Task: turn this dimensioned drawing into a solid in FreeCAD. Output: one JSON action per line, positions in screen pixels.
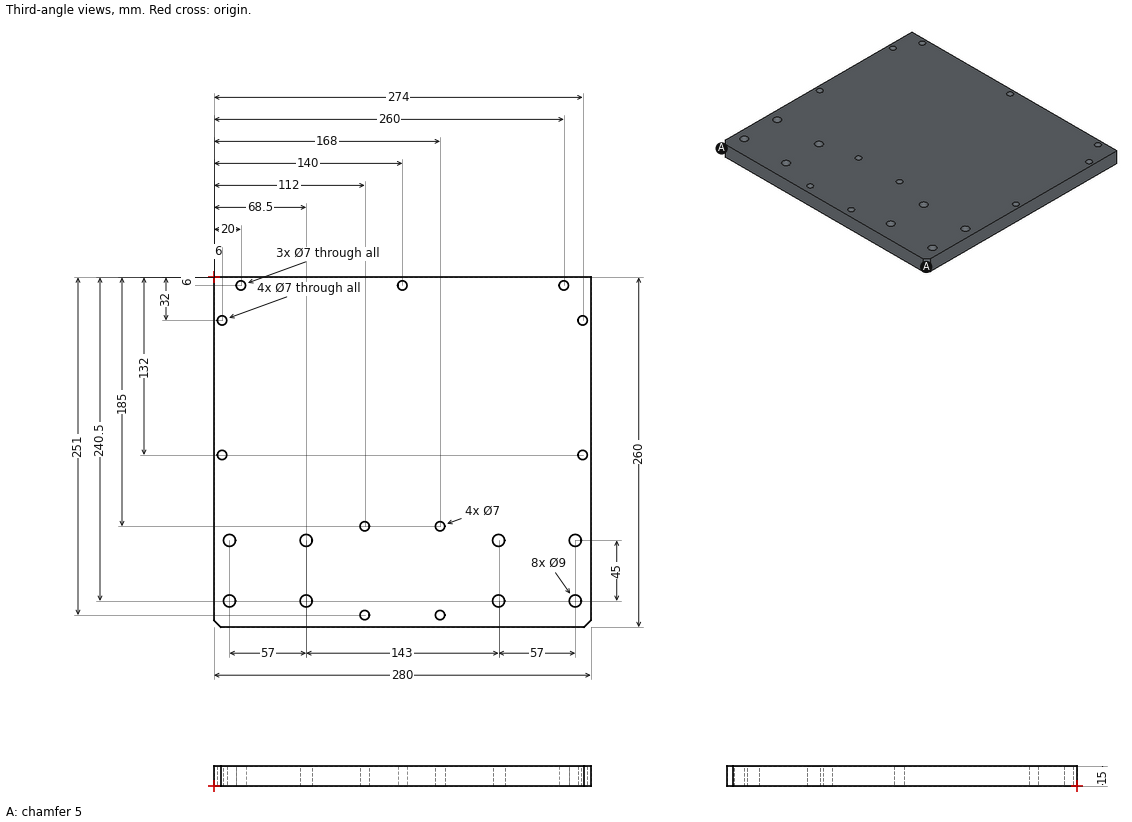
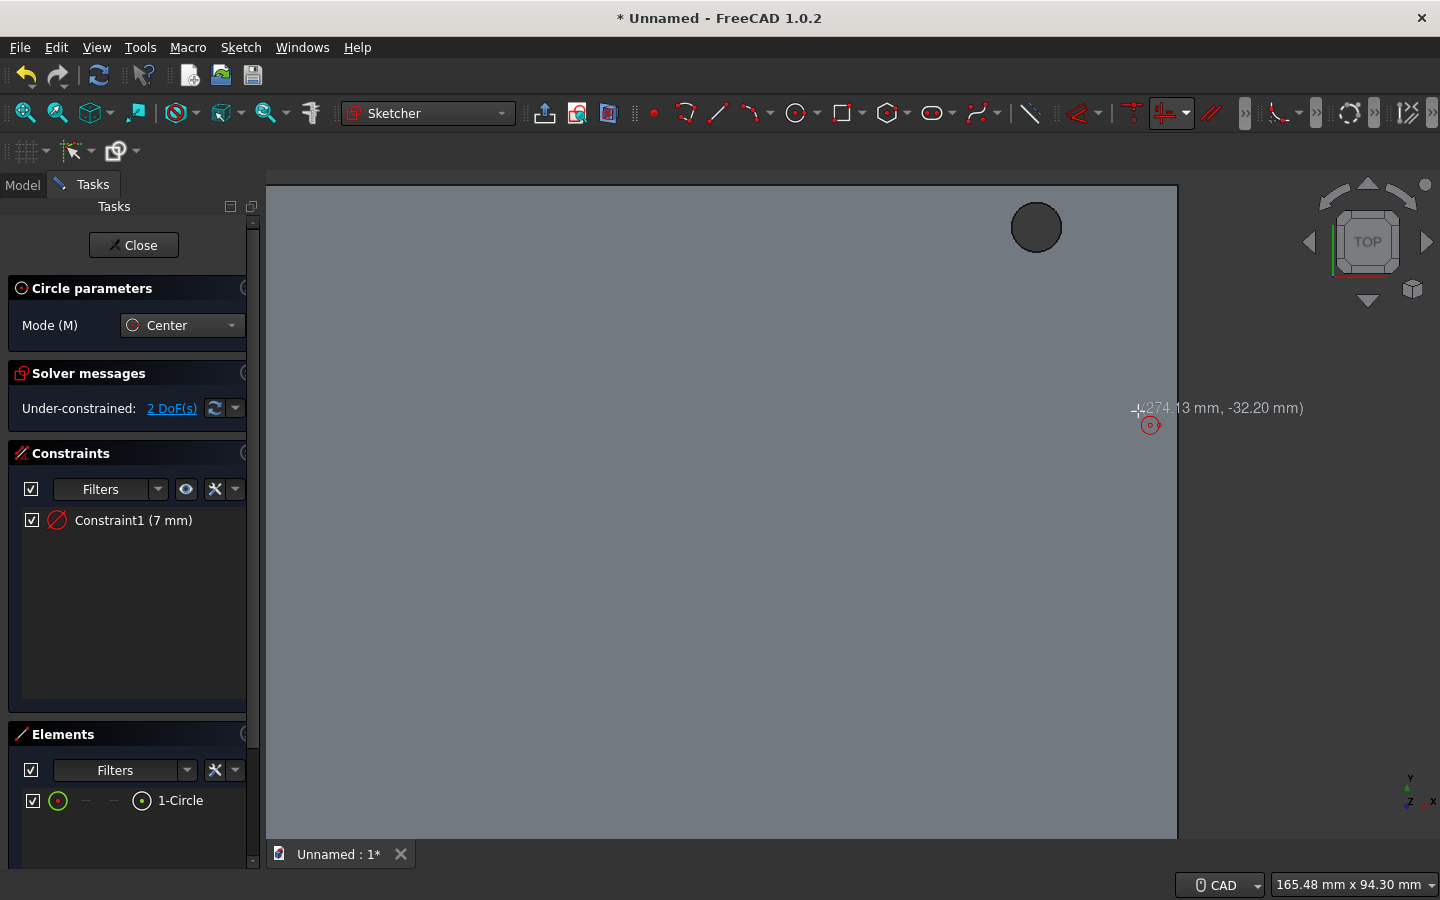
{"action": "left_click", "coordinate": [1136, 412]}
{"action": "mouse_move", "coordinate": [1153, 394]}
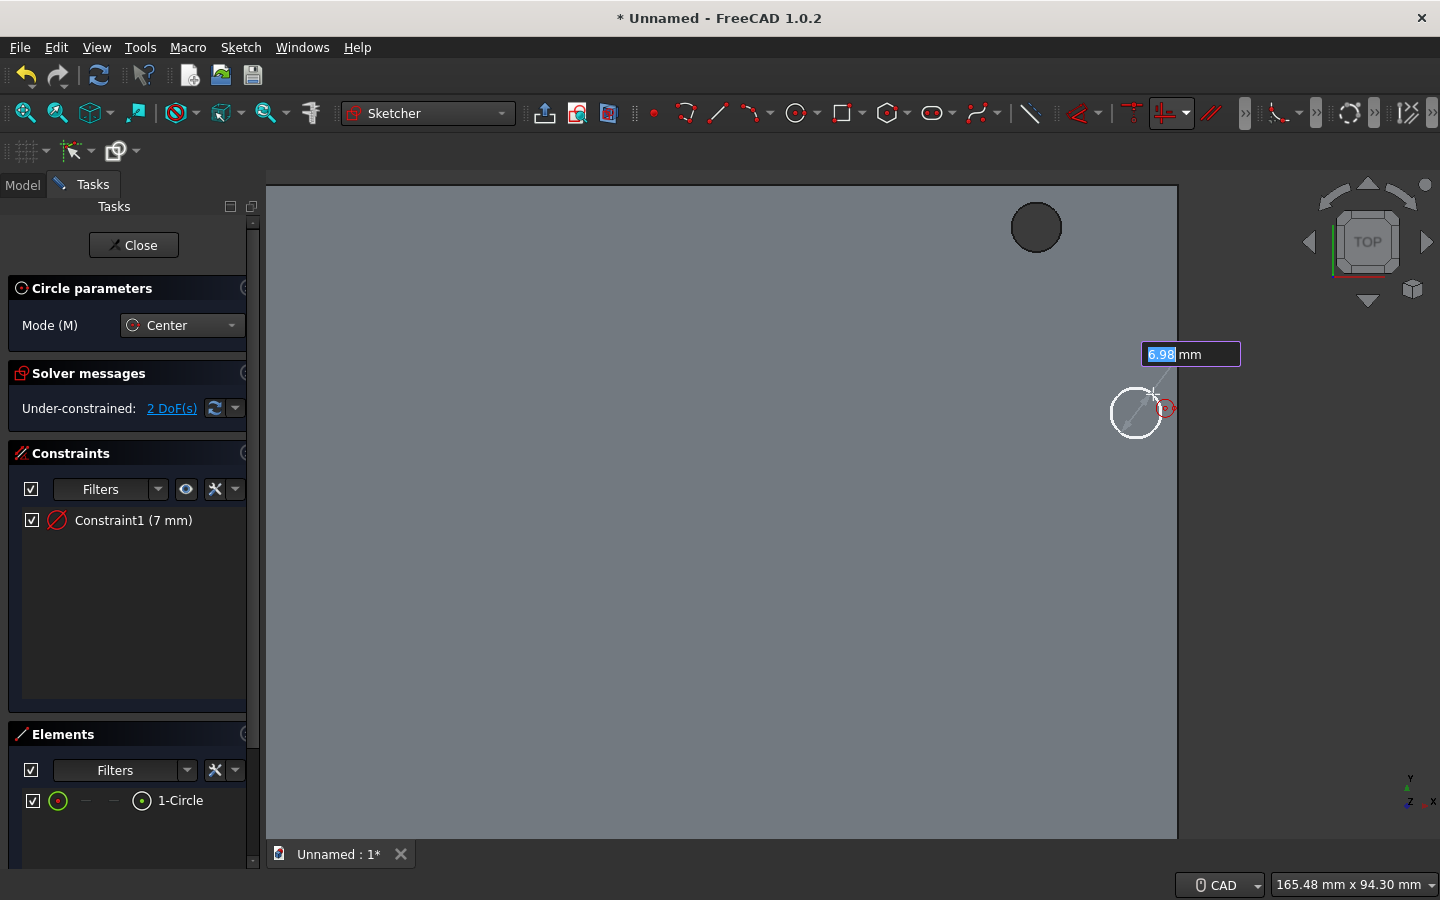
{"action": "type", "text": "7"}
{"action": "key", "text": "Return"}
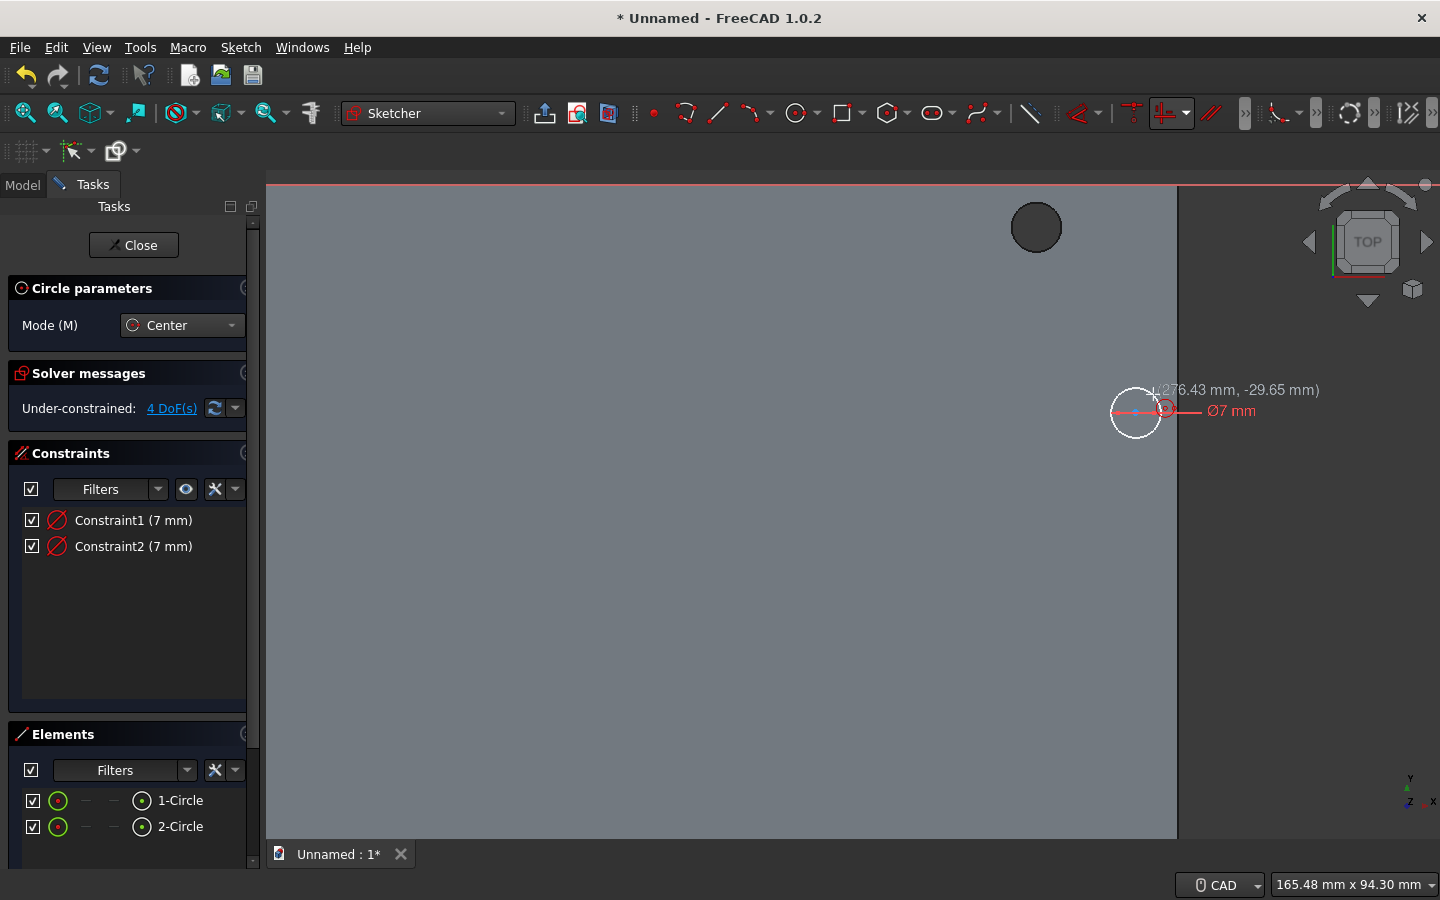
{"action": "scroll", "coordinate": [1138, 411], "scroll_direction": "down", "scroll_amount": 5}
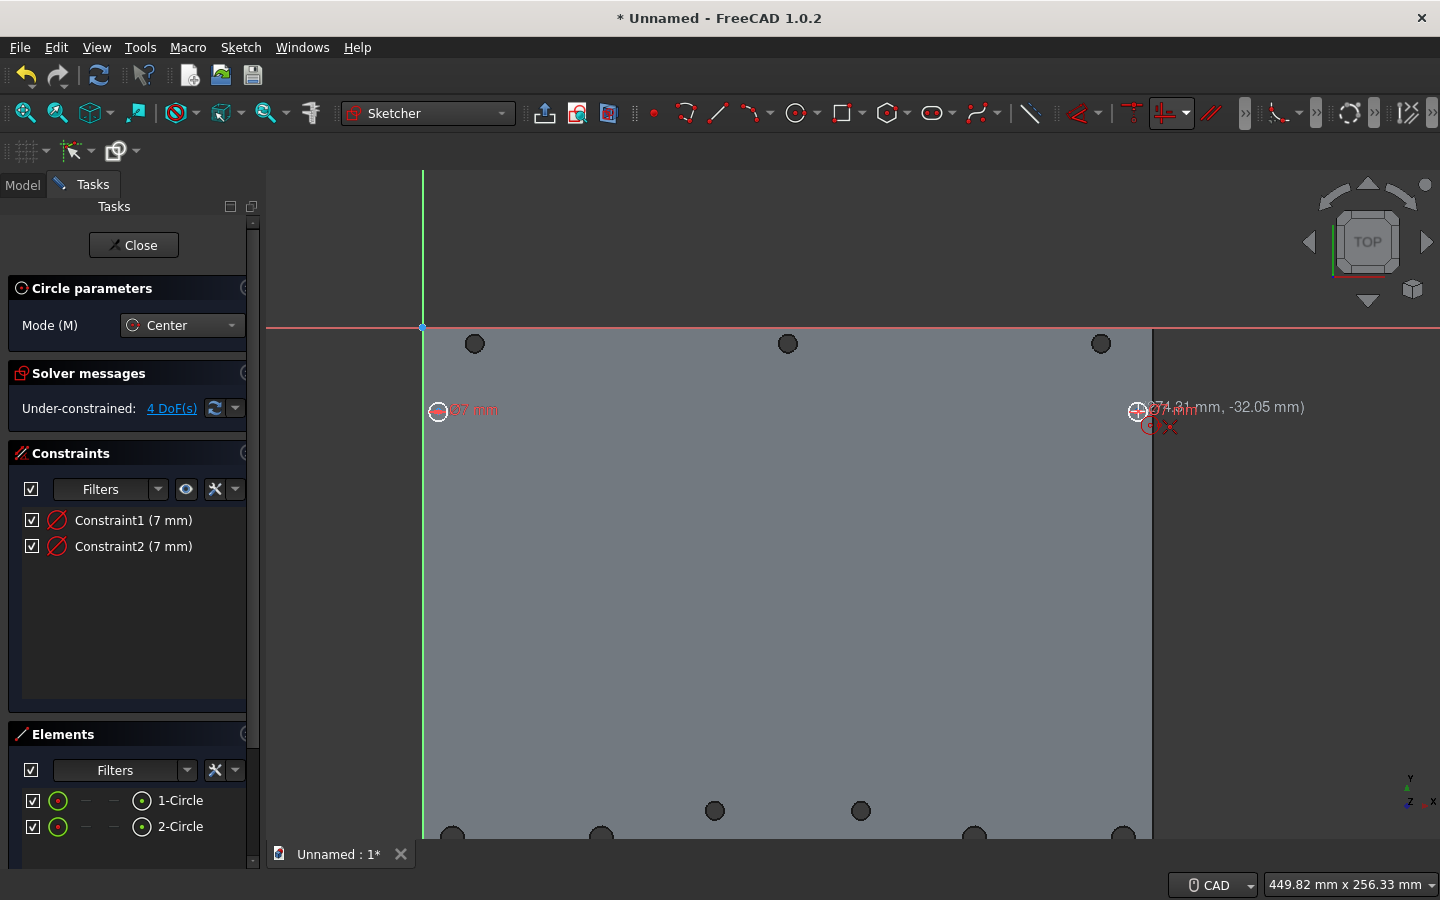
{"action": "scroll", "coordinate": [1138, 672], "scroll_direction": "up", "scroll_amount": 5}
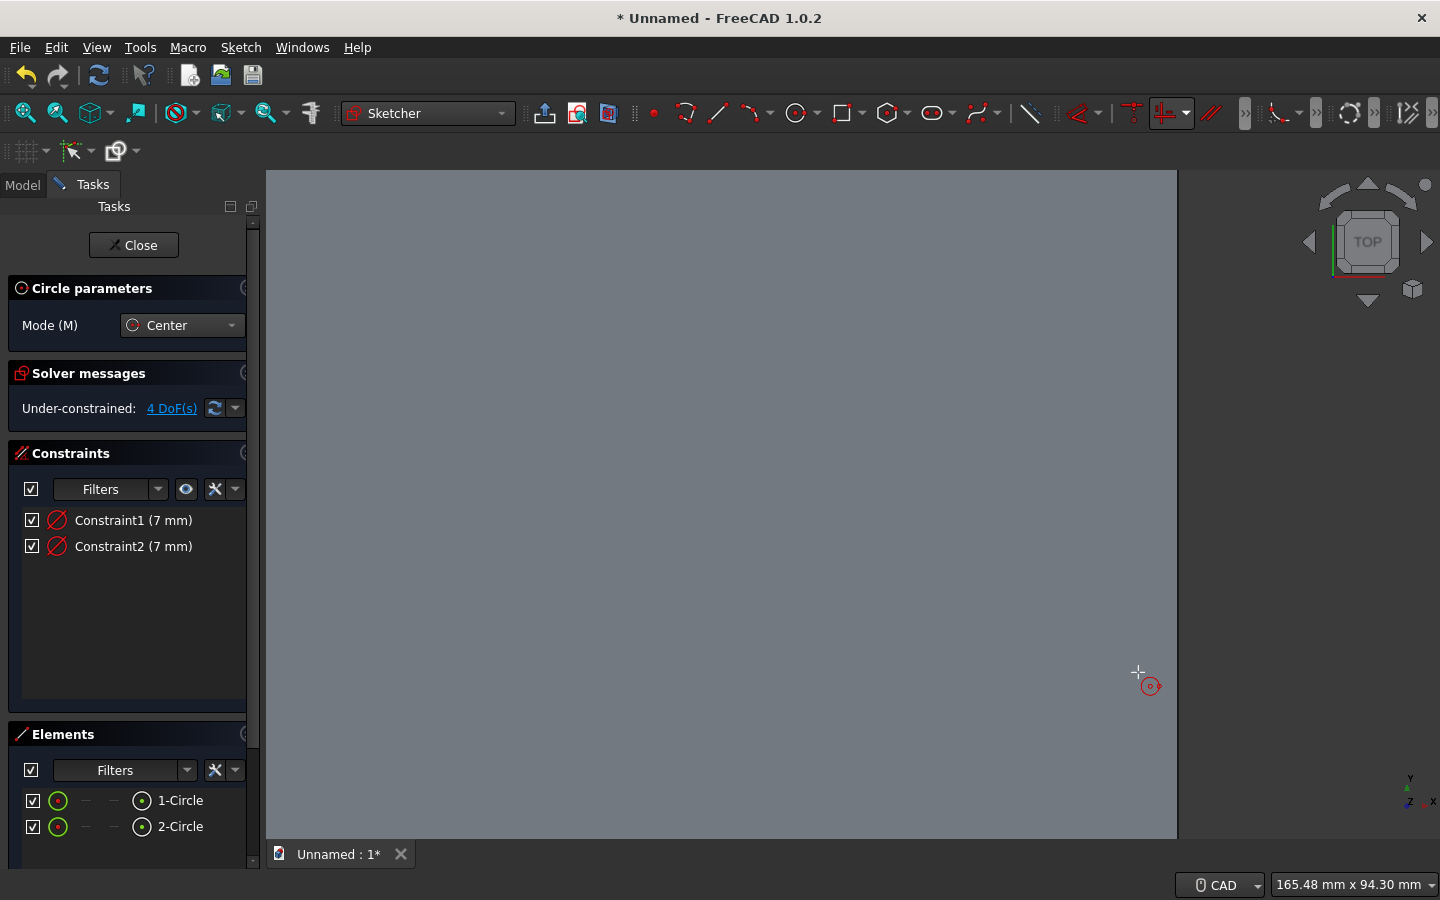
{"action": "left_click", "coordinate": [1136, 672]}
{"action": "mouse_move", "coordinate": [1153, 654]}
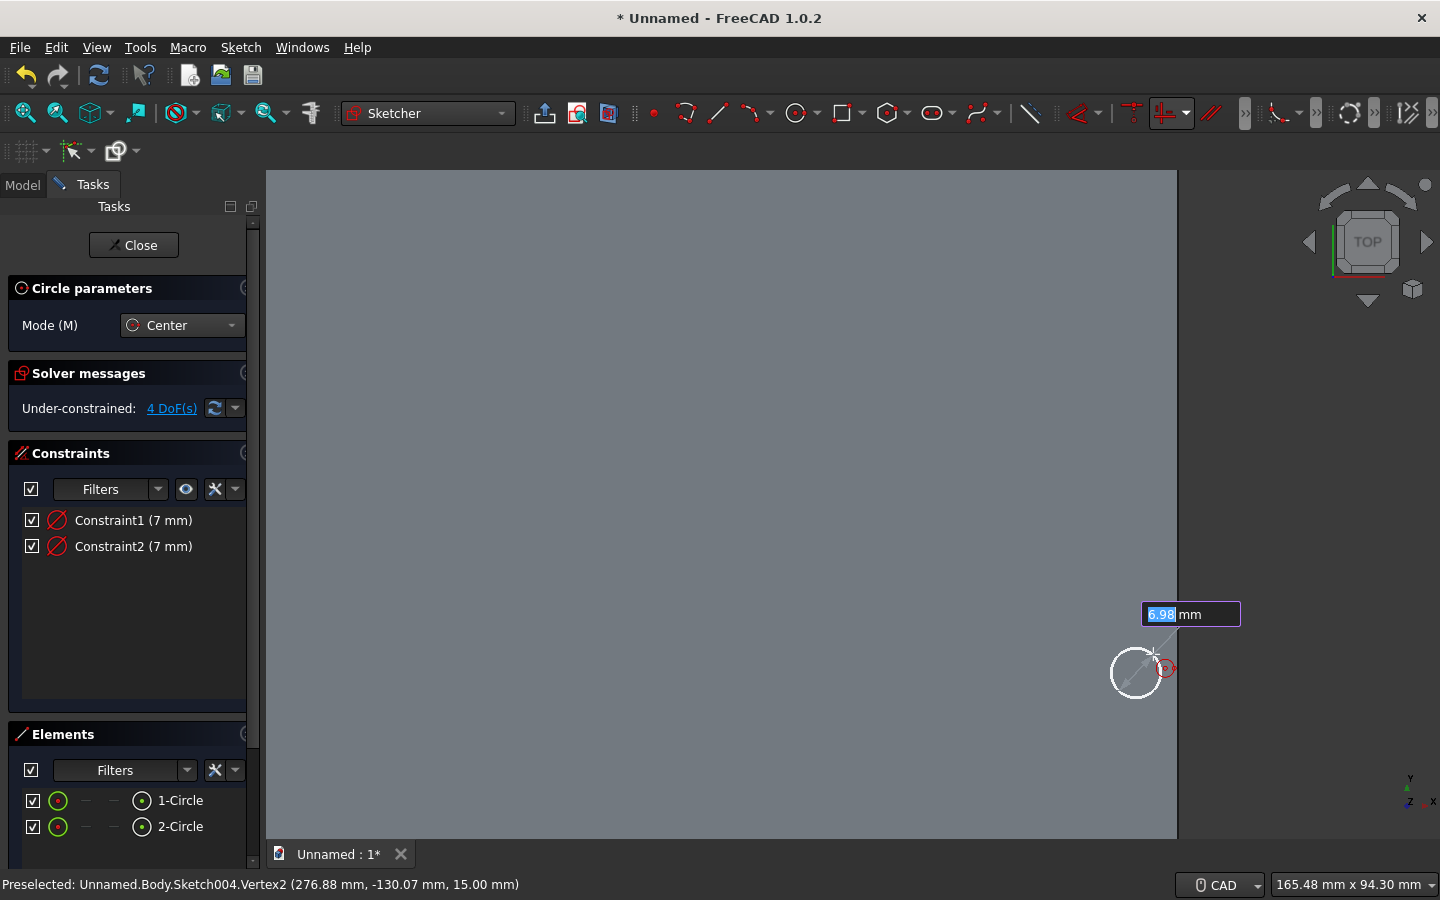
{"action": "type", "text": "7"}
{"action": "key", "text": "Return"}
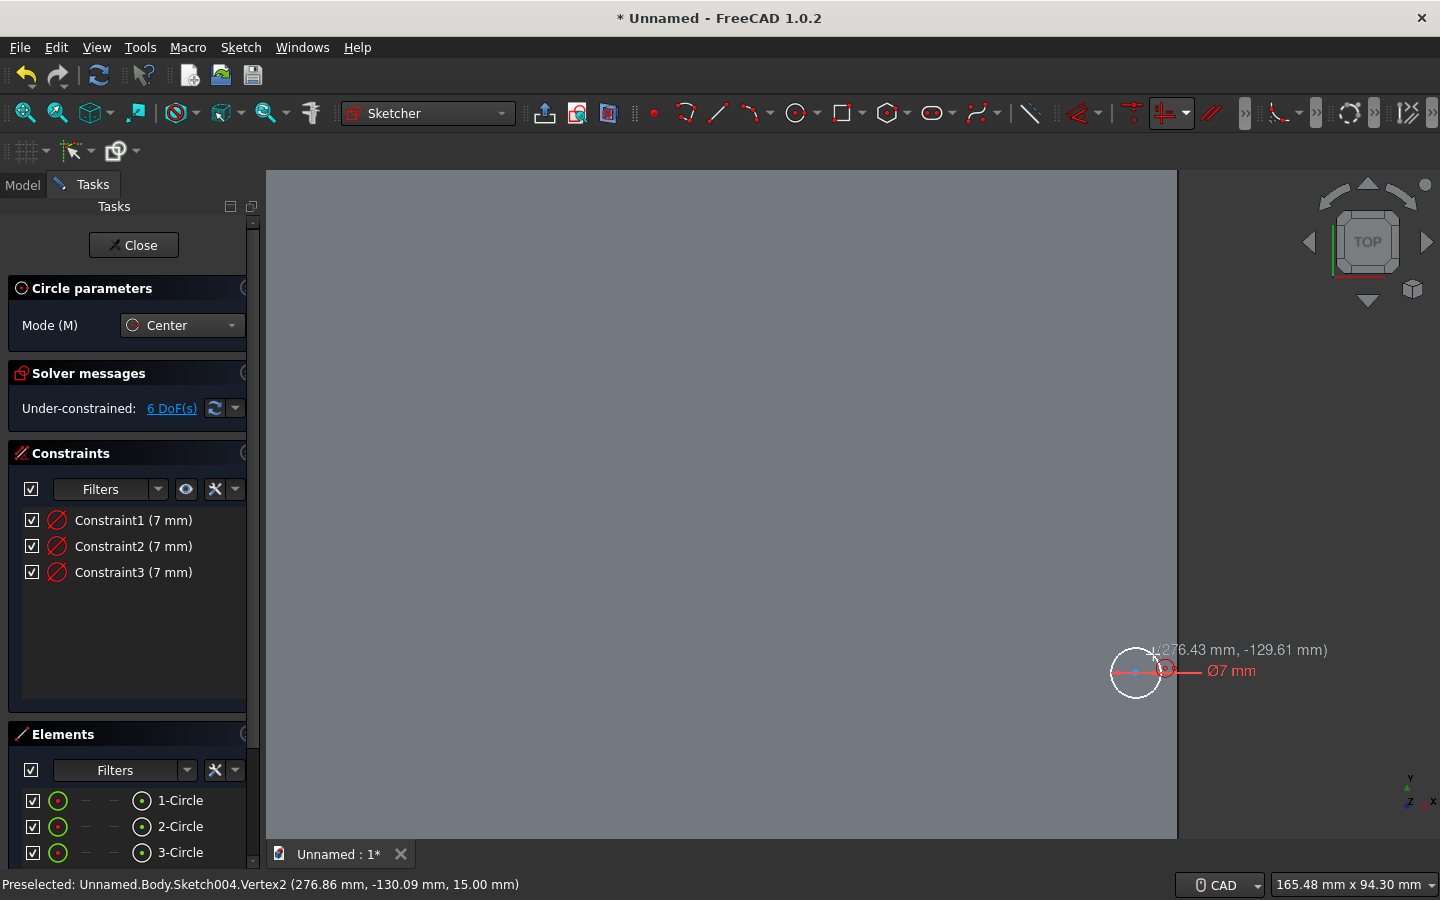
{"action": "scroll", "coordinate": [1138, 672], "scroll_direction": "down", "scroll_amount": 5}